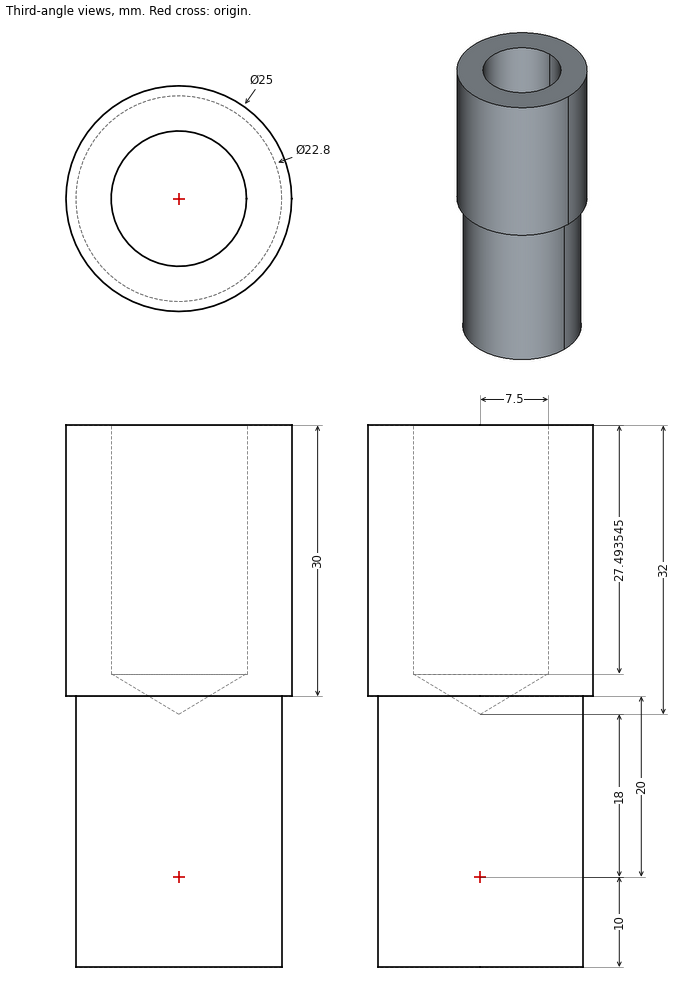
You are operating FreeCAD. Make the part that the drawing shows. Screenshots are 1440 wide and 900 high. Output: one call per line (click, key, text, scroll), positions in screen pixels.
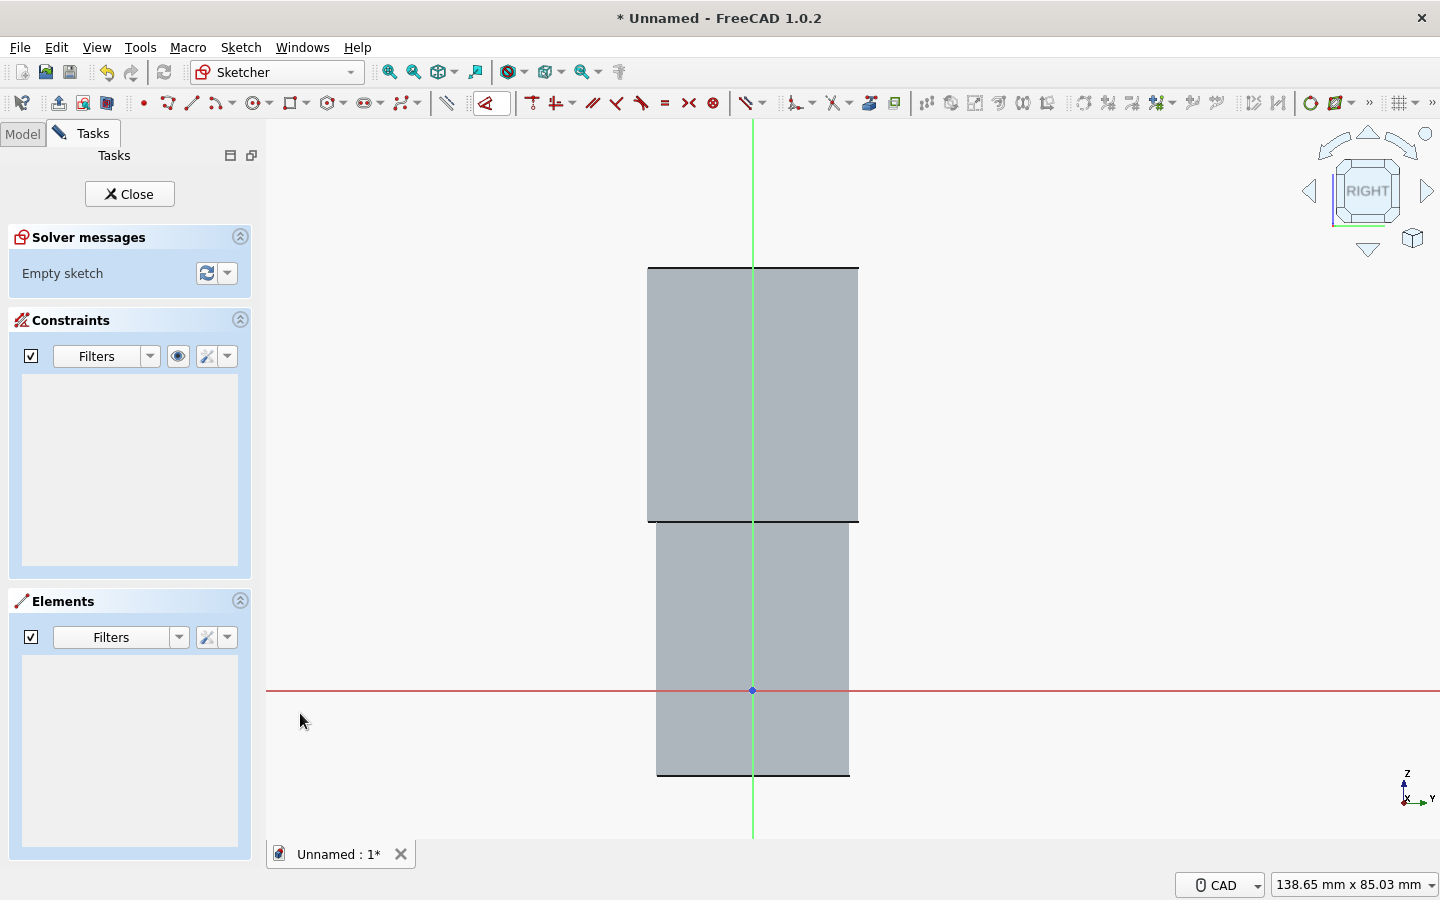
click(168, 104)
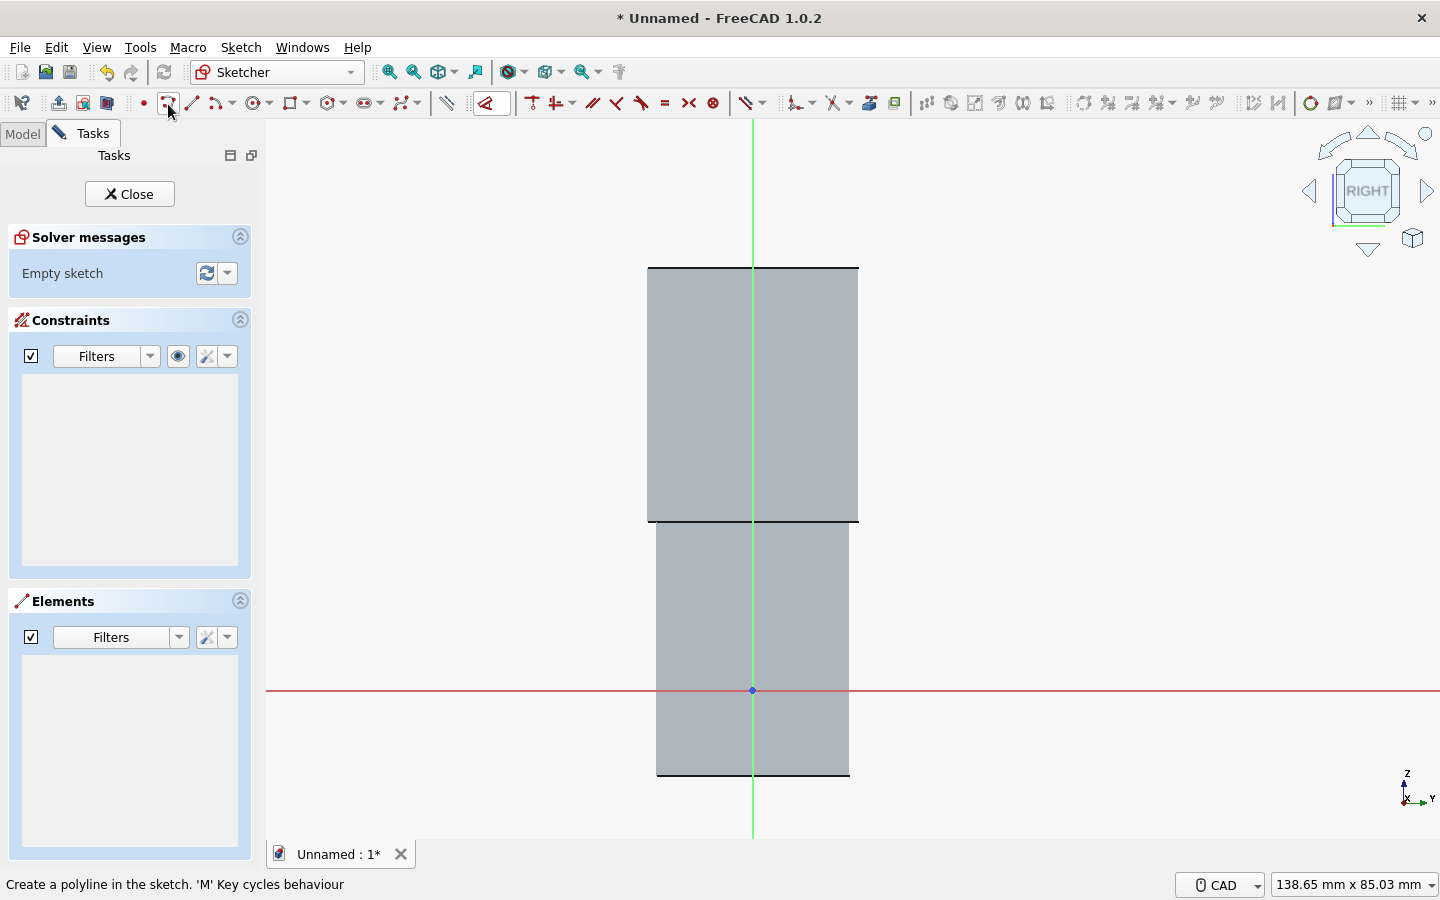
click(753, 539)
click(816, 500)
click(816, 268)
click(762, 268)
click(753, 540)
key(Escape)
key(Escape)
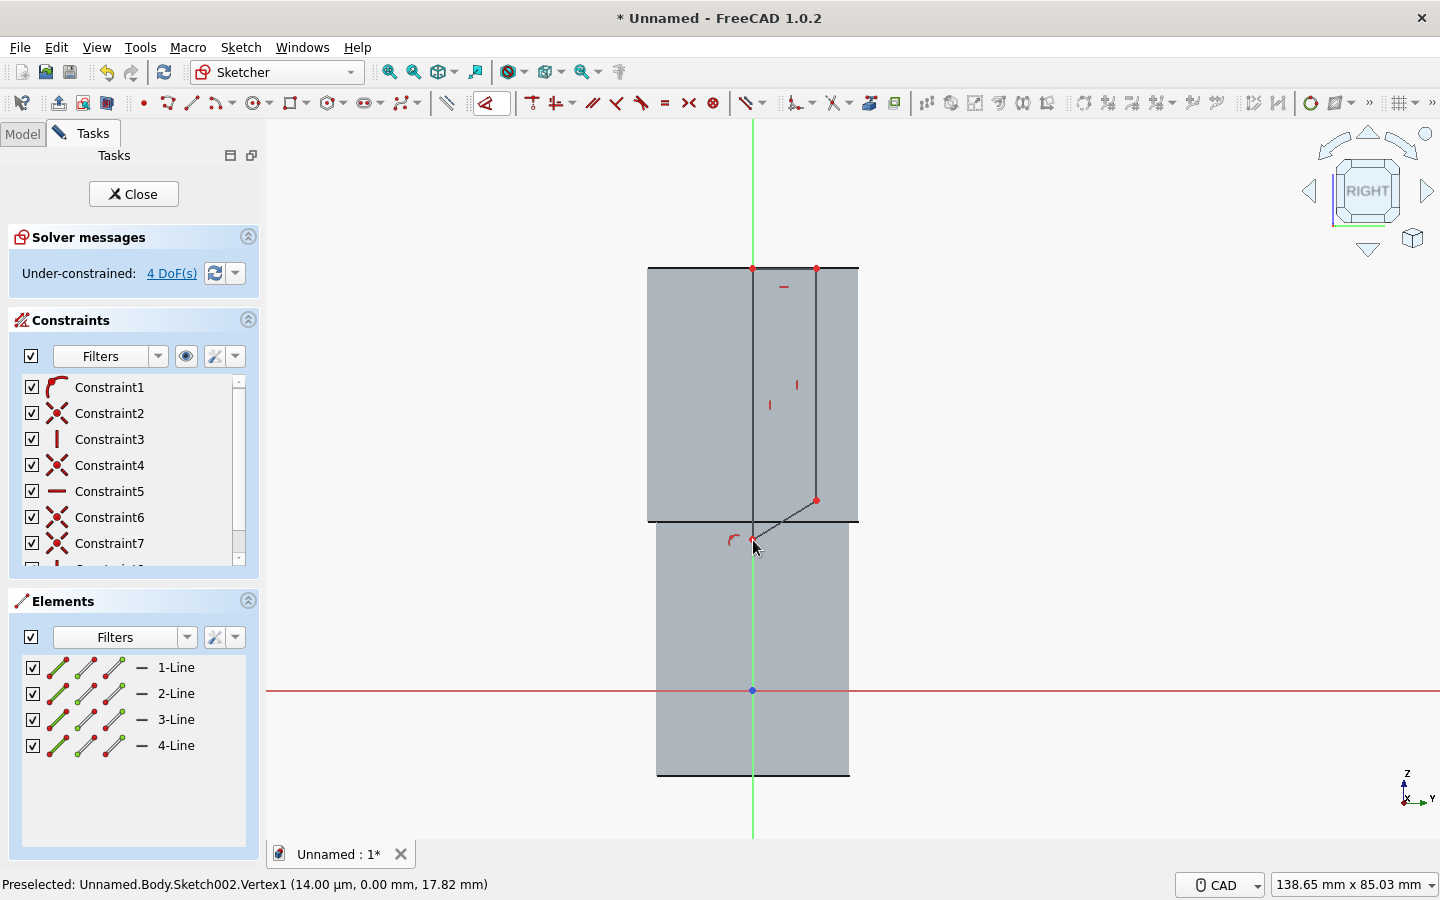
key(d)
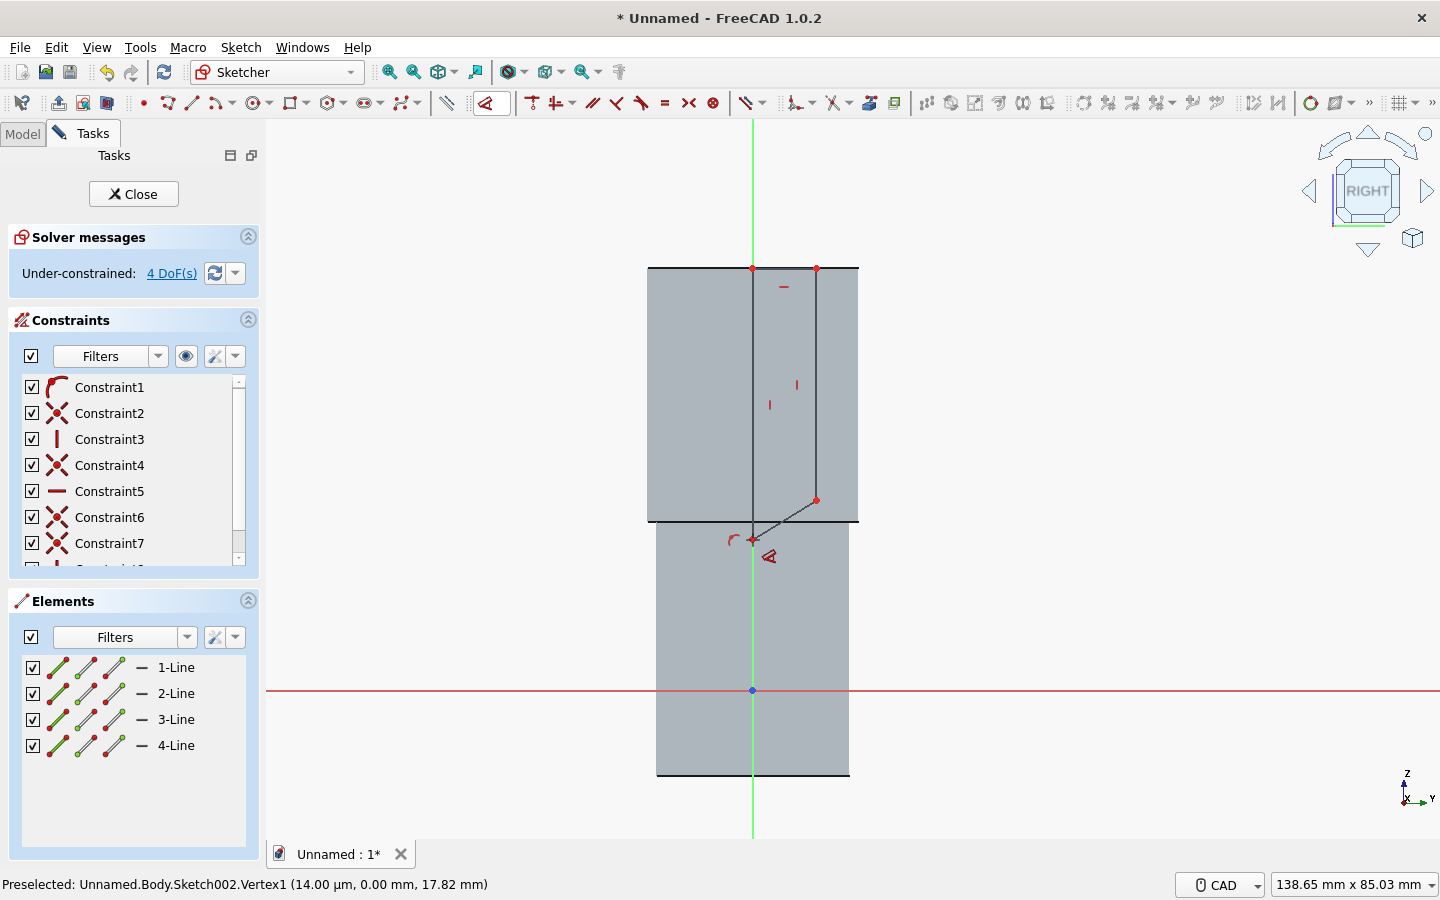
click(753, 350)
click(719, 405)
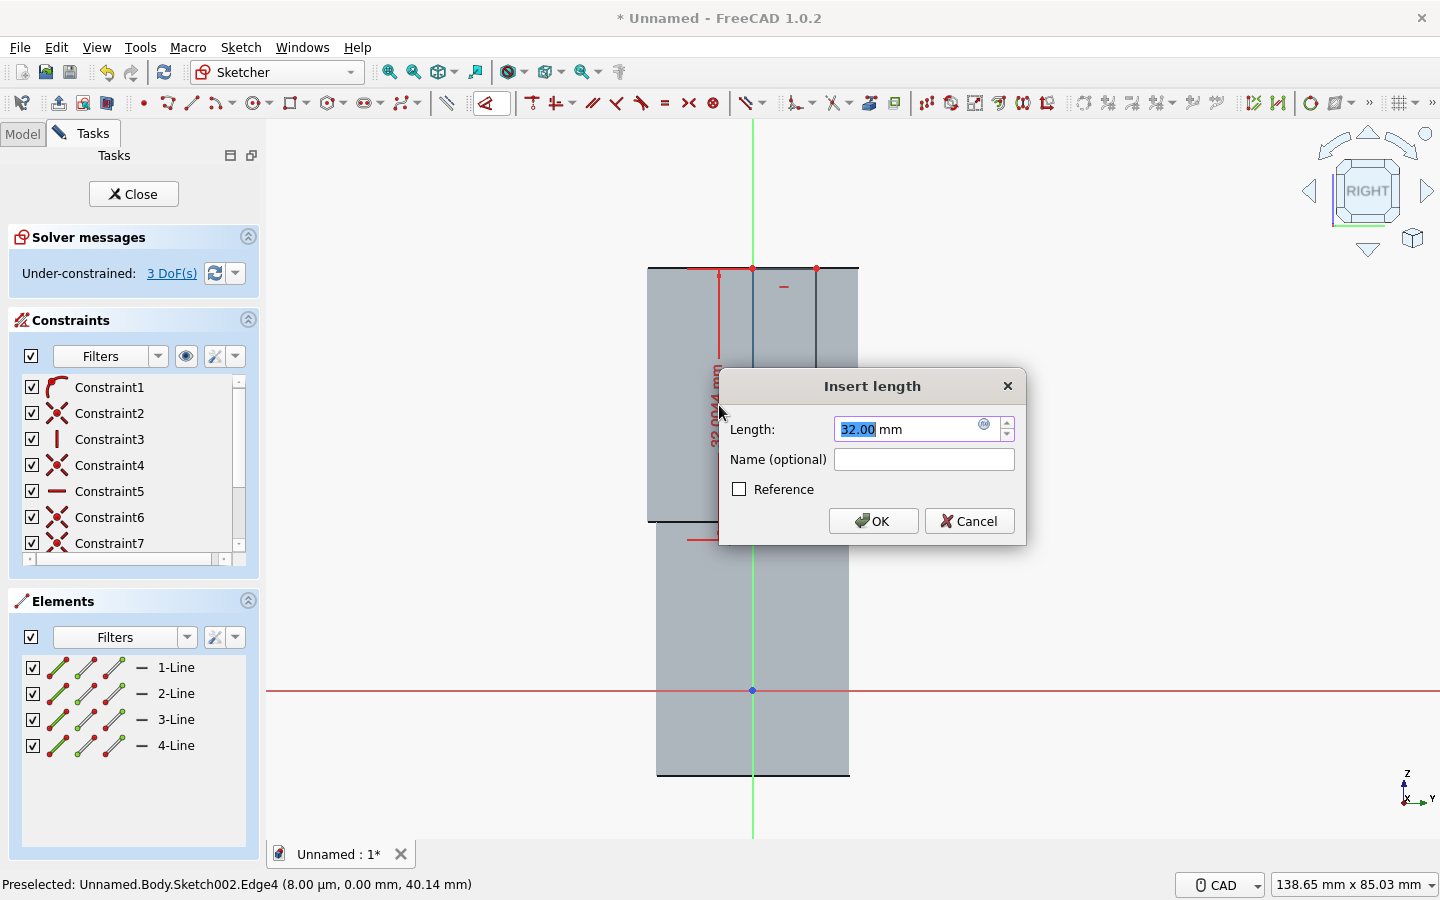
text(32)
key(Return)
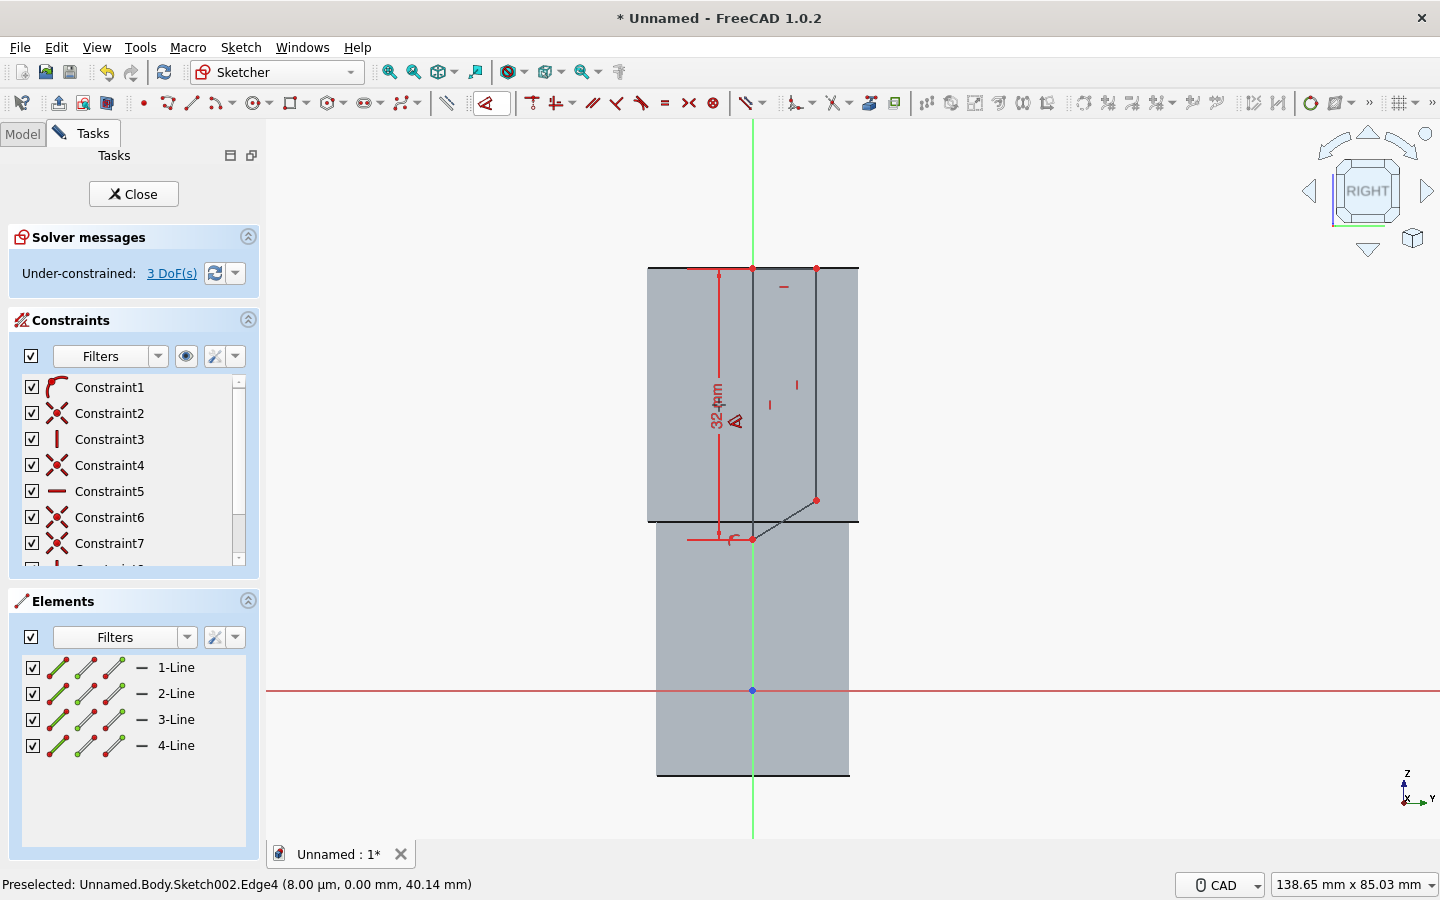
click(797, 269)
click(784, 235)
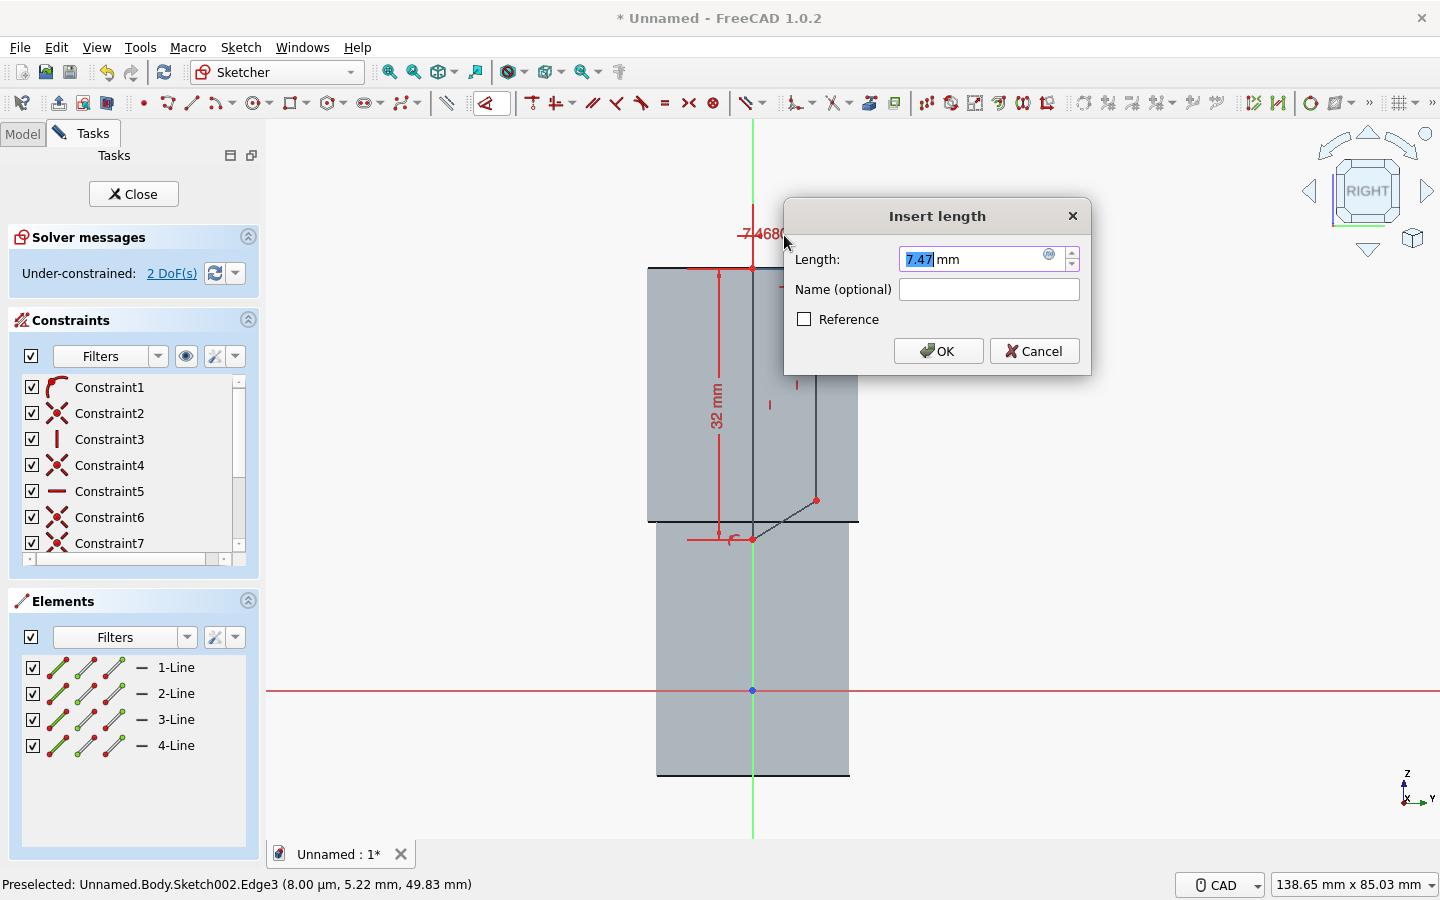
text(7.5)
key(Return)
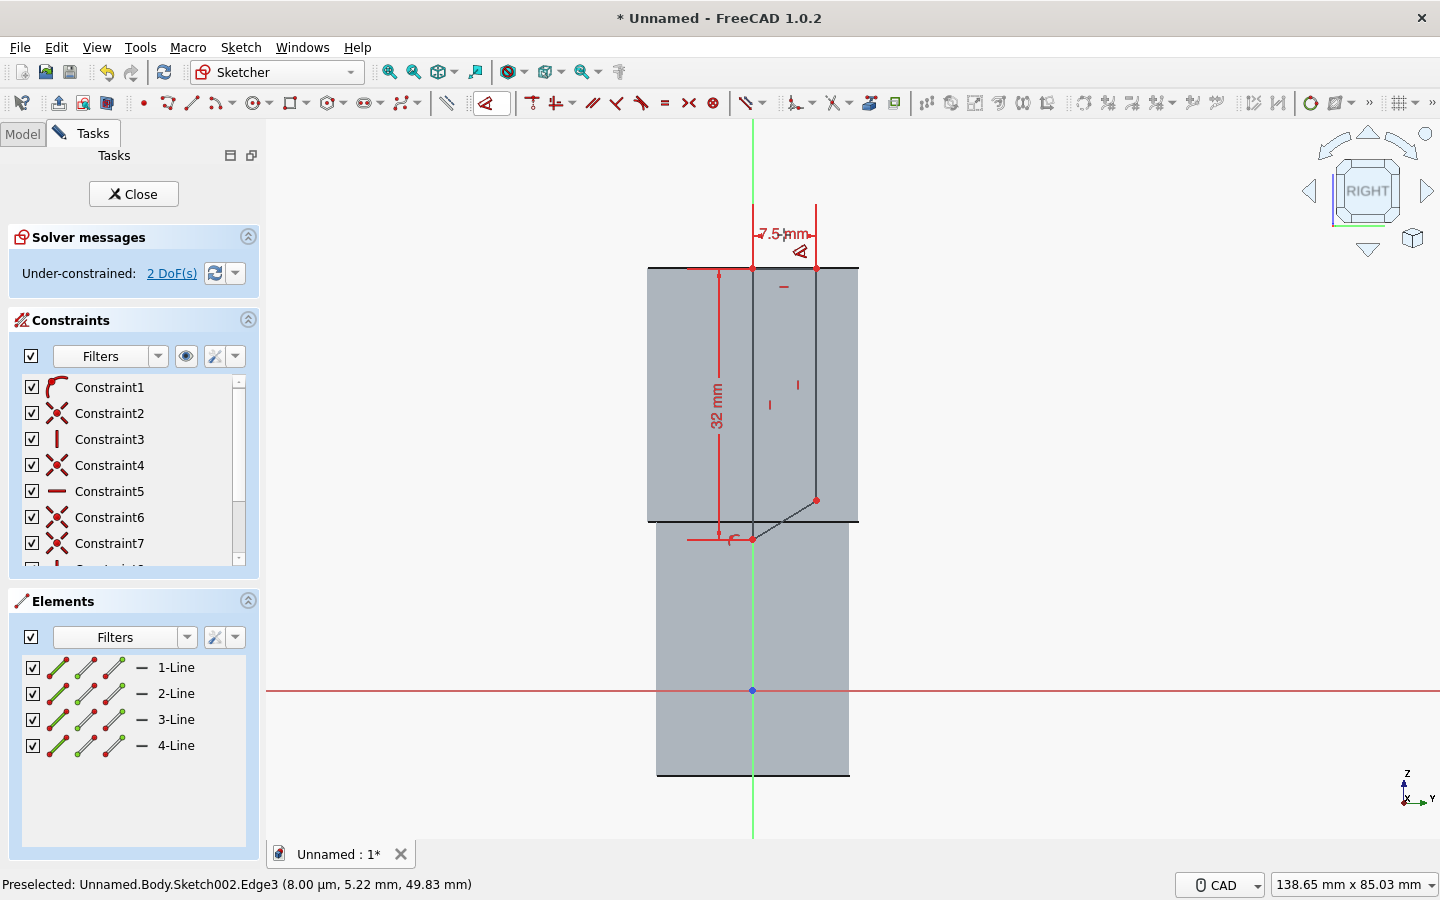
click(753, 540)
click(719, 615)